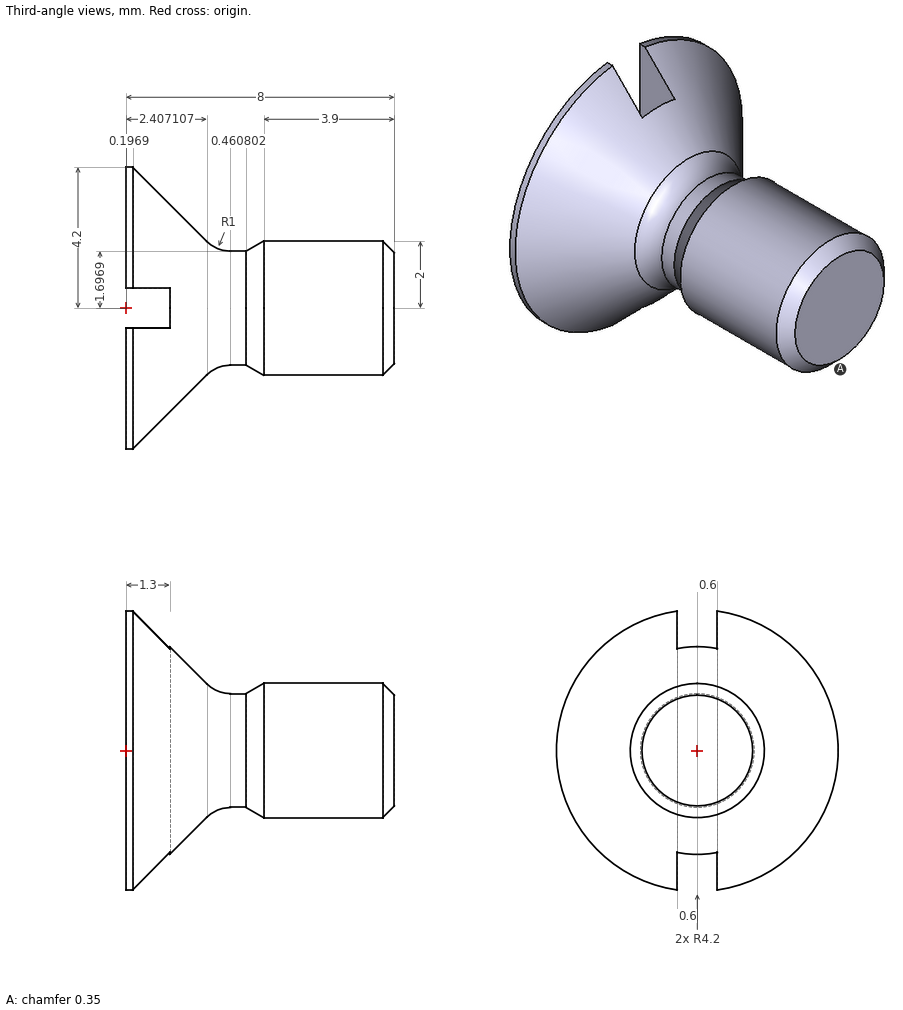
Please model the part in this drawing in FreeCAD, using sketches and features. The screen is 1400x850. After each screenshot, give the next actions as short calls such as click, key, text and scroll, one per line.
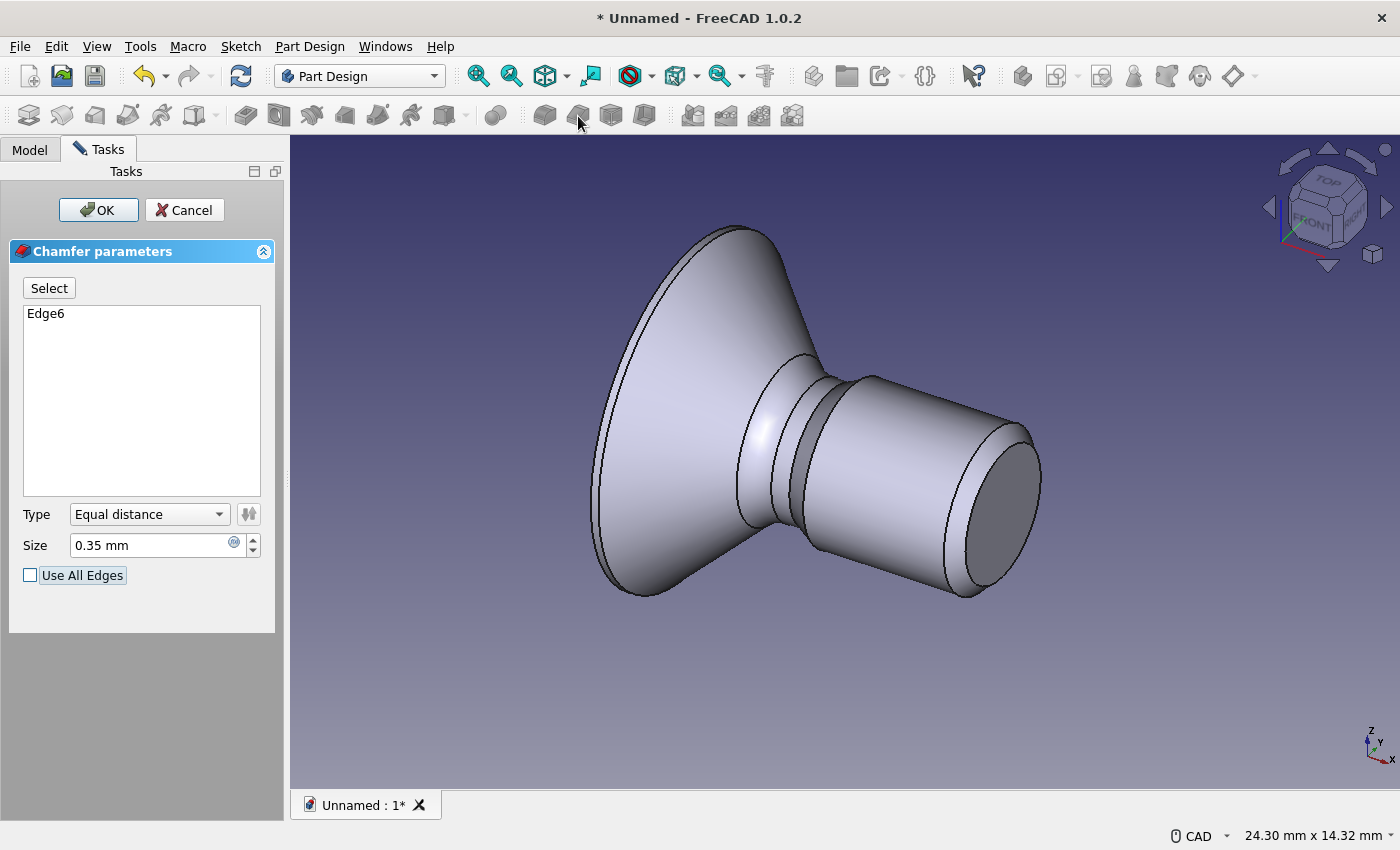
click(99, 210)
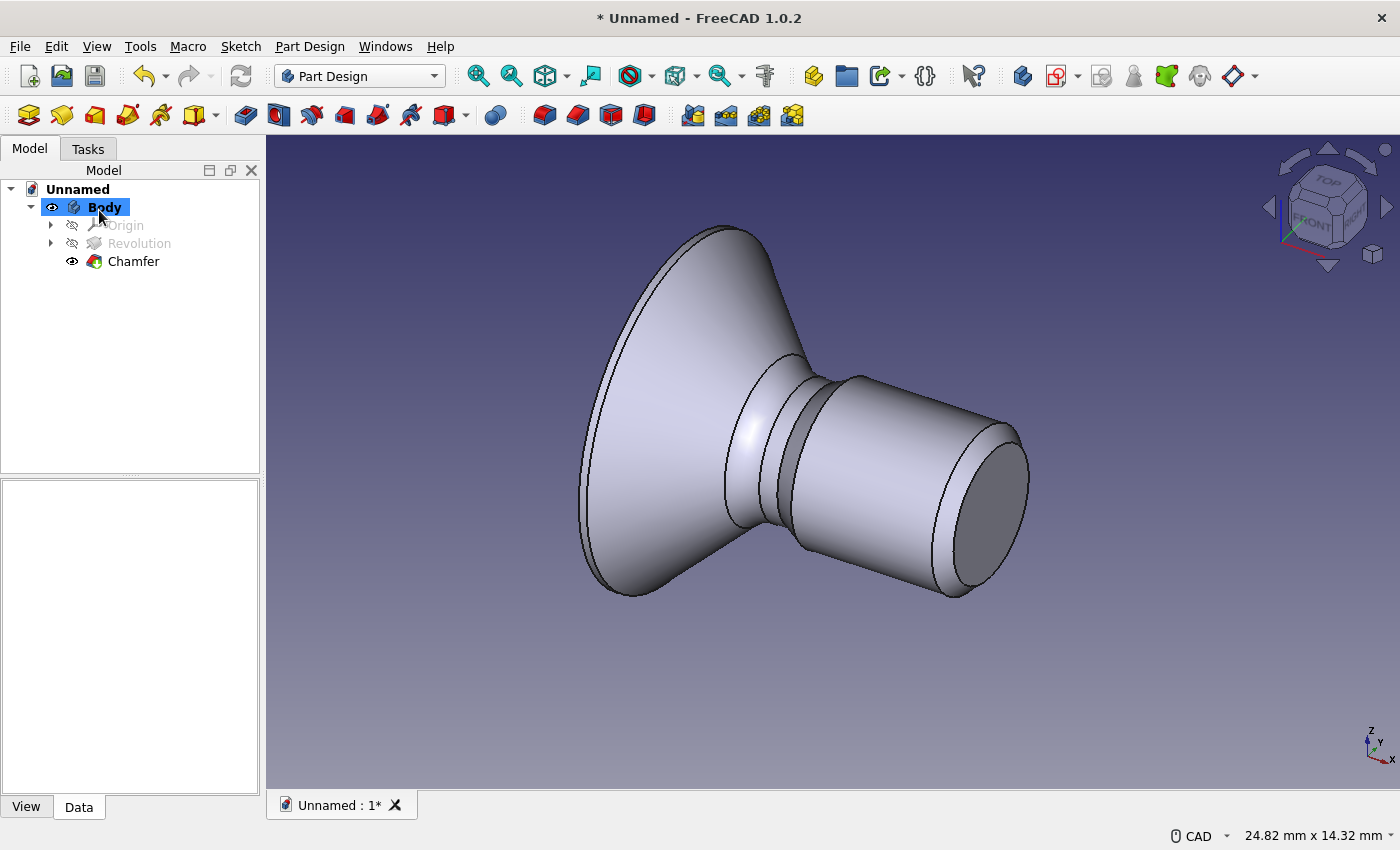
click(51, 225)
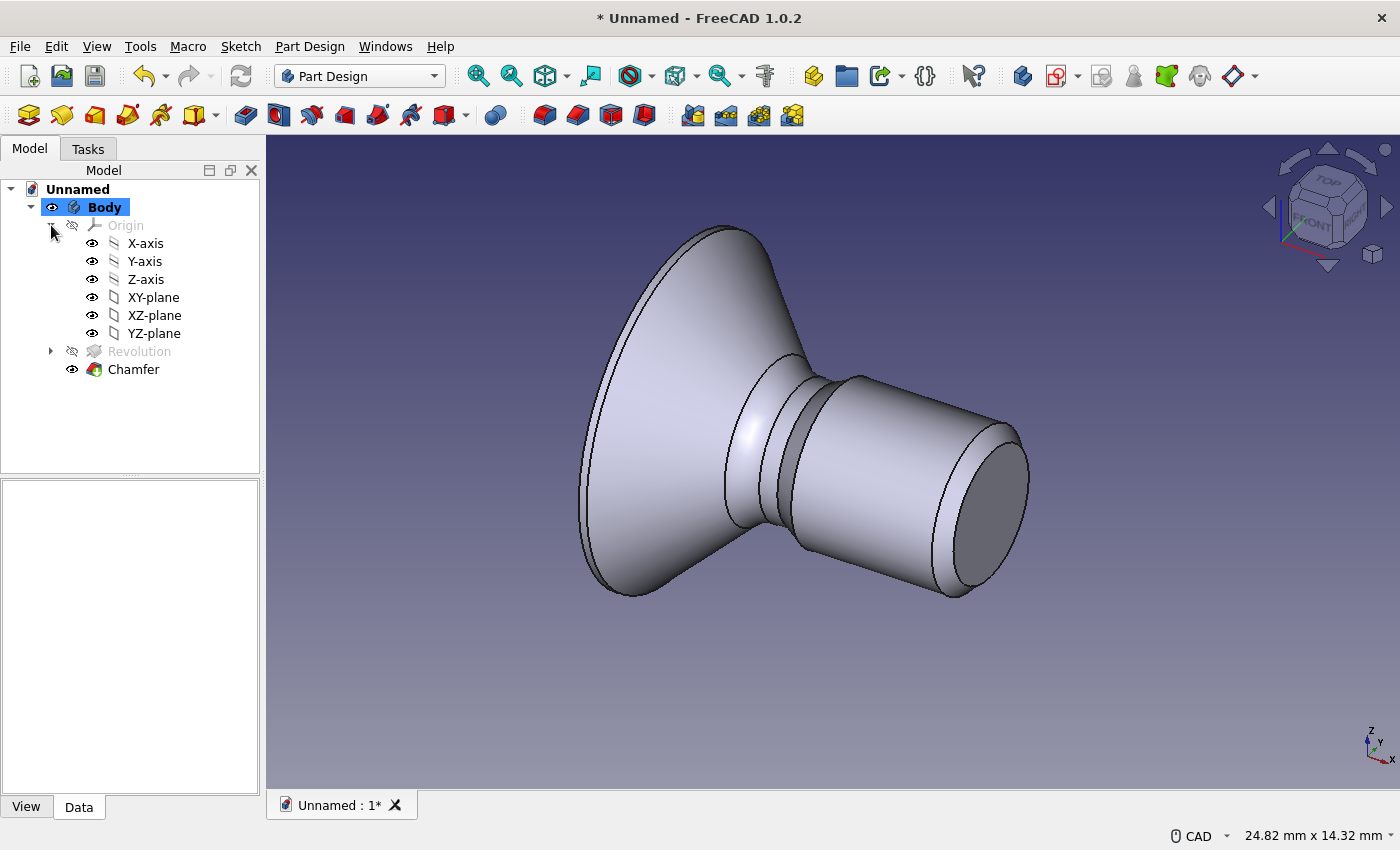
click(137, 333)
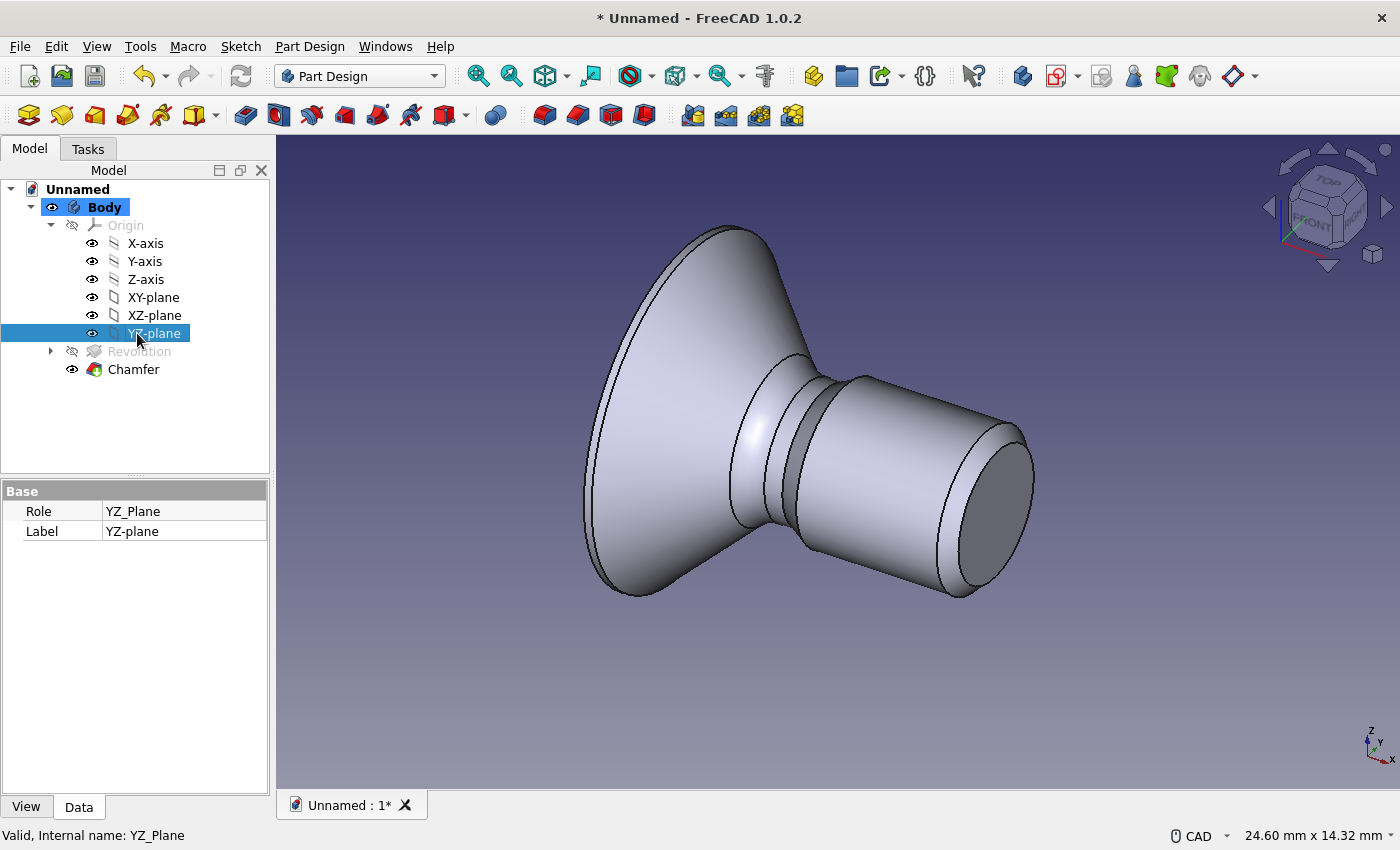
click(1232, 76)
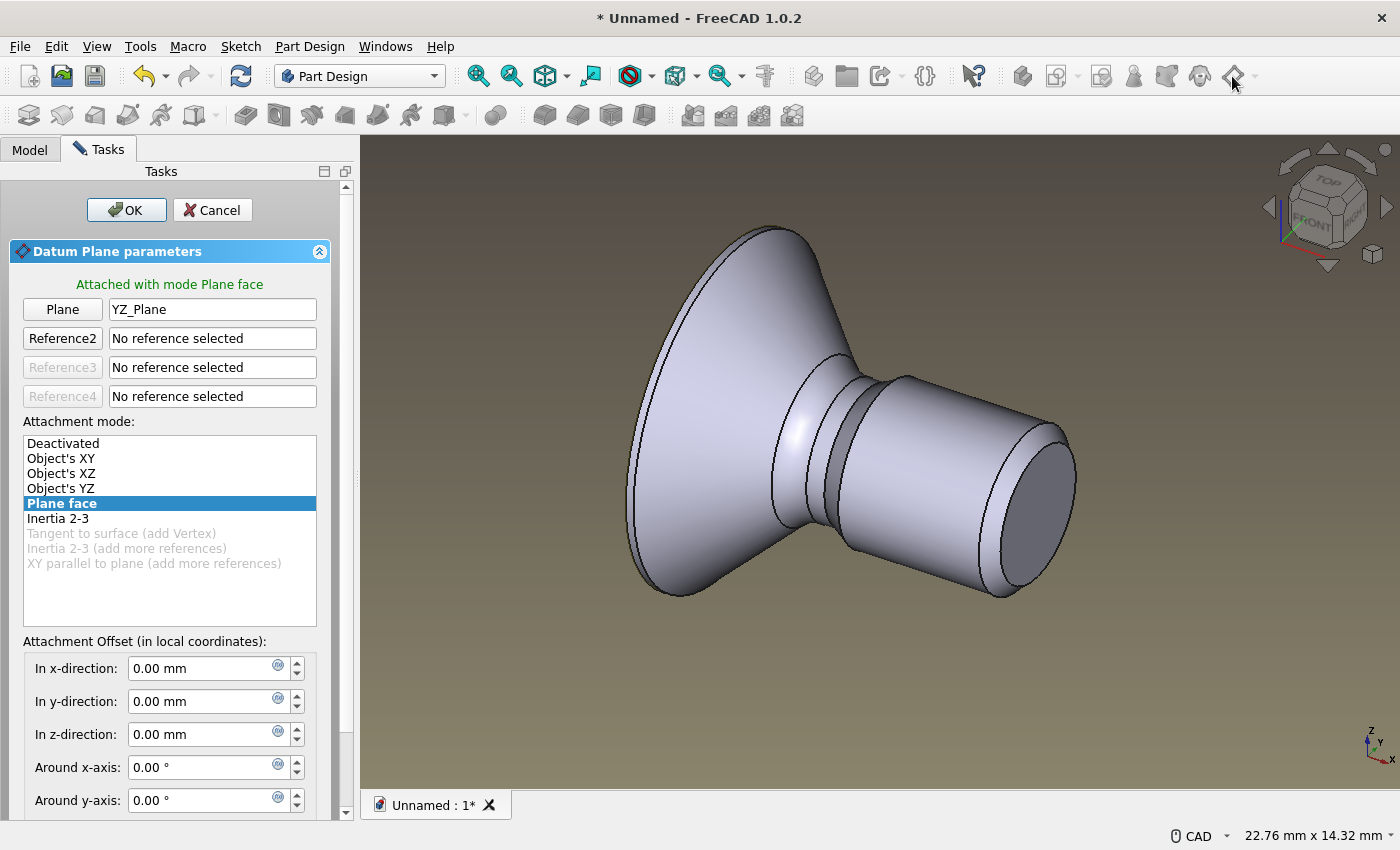
triple_click(210, 734)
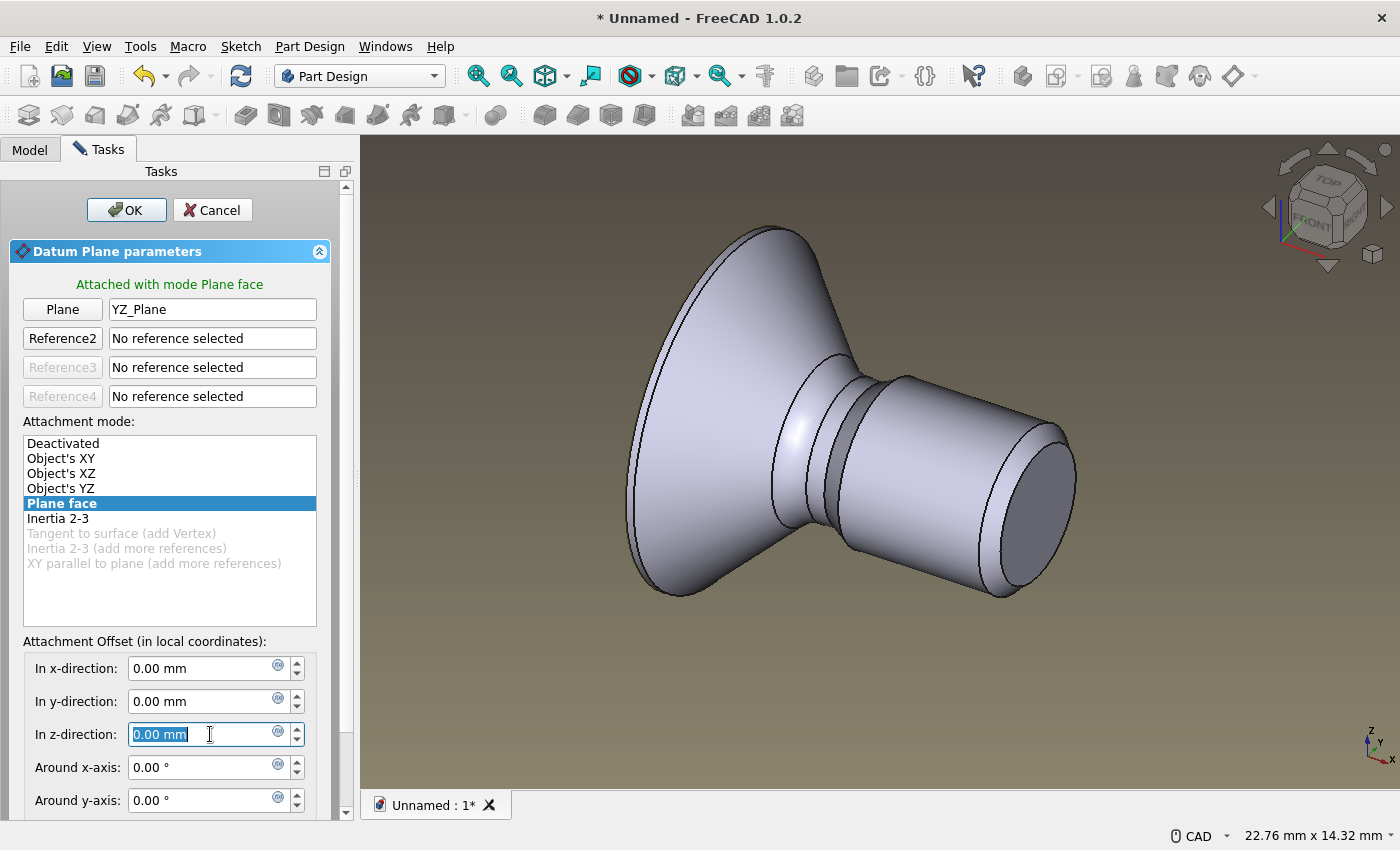
text(1.3)
key(Tab)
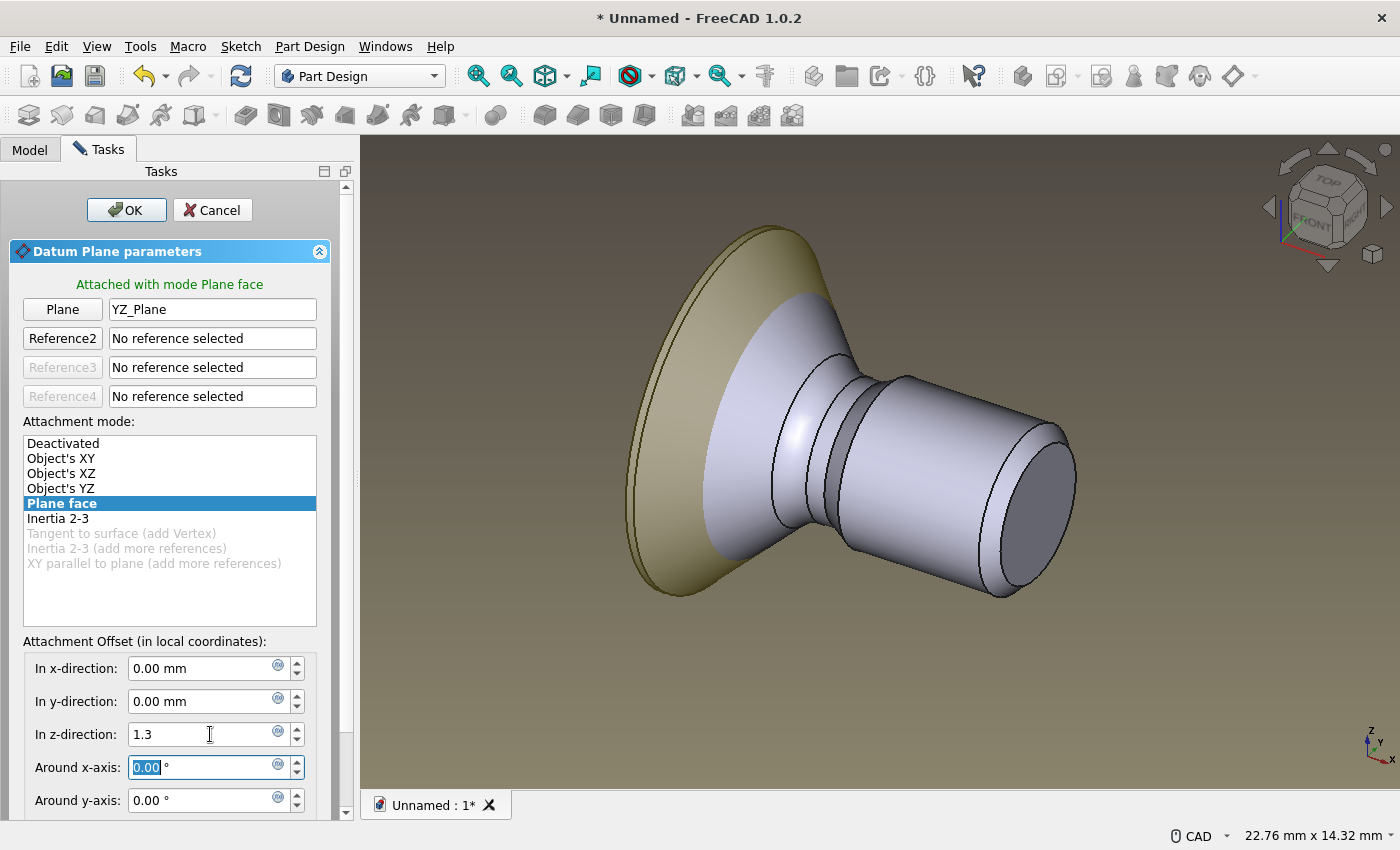
click(127, 210)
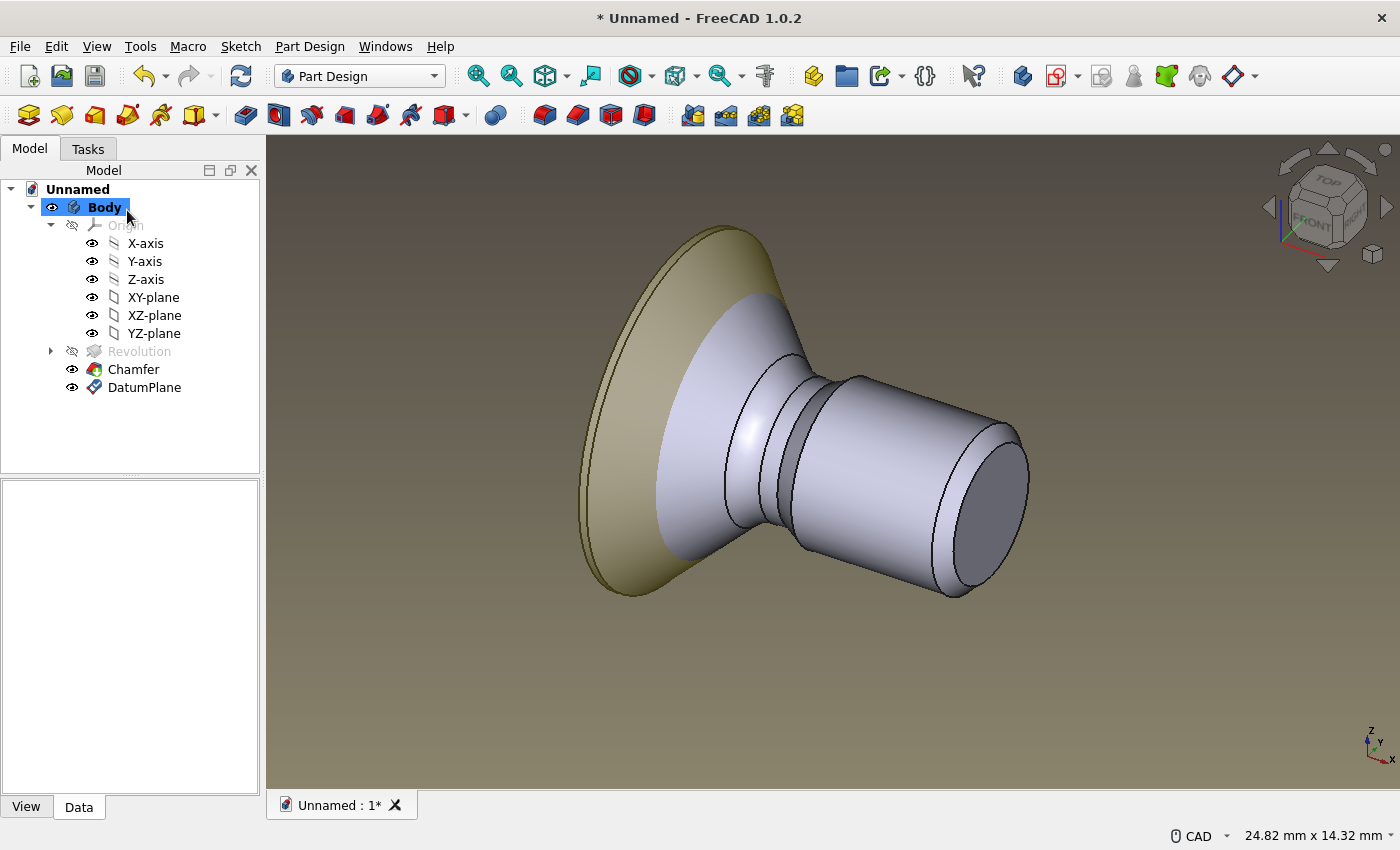
click(117, 387)